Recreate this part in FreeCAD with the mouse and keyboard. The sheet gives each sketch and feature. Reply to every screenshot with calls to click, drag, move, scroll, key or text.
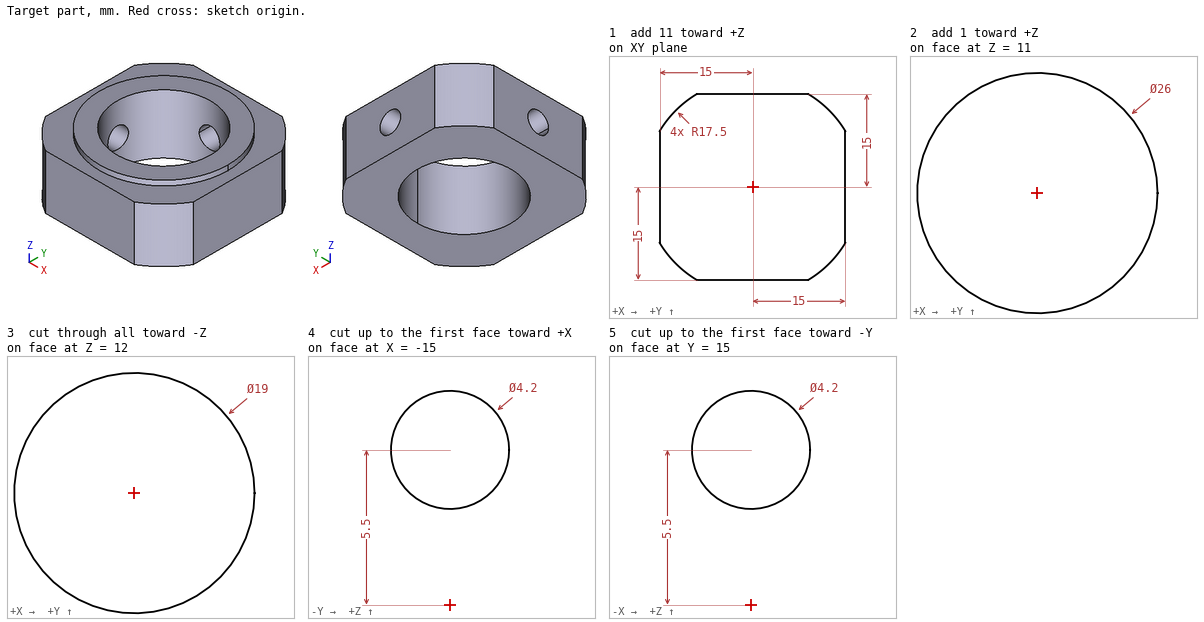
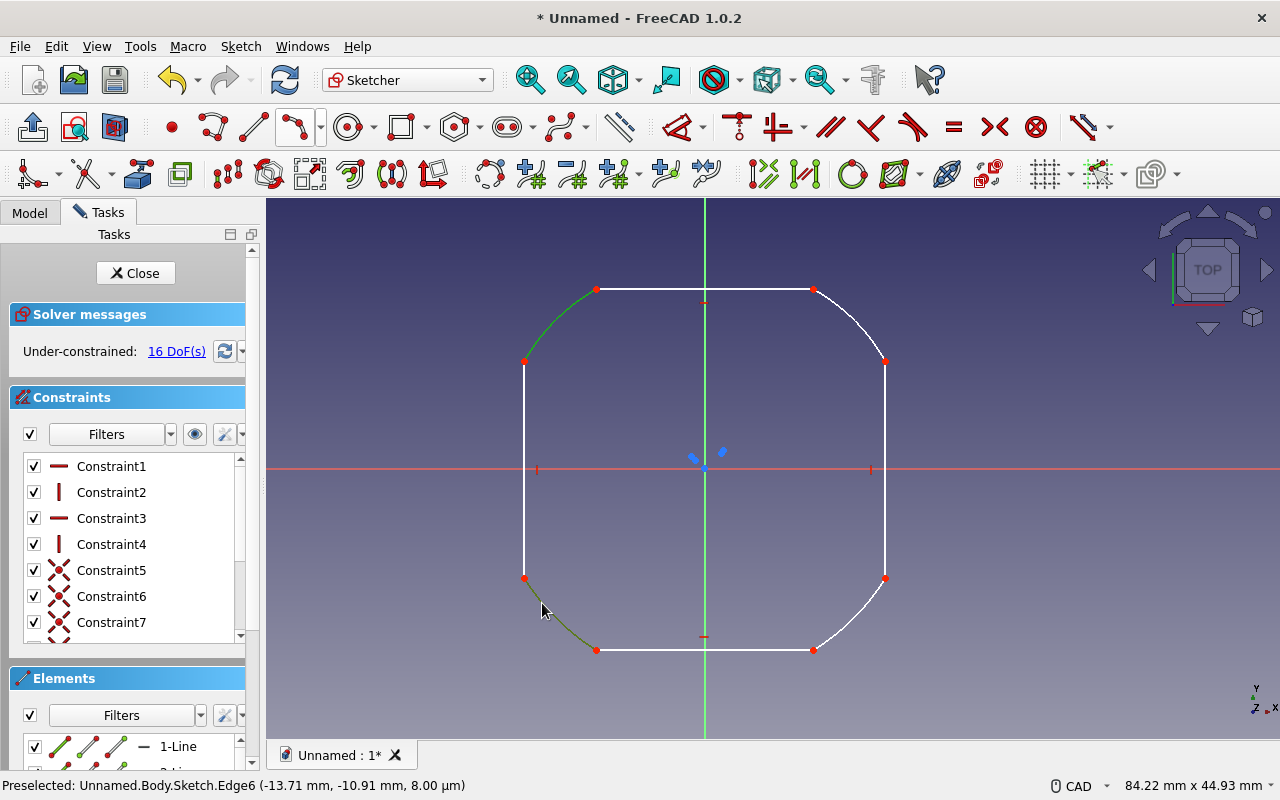
click(737, 128)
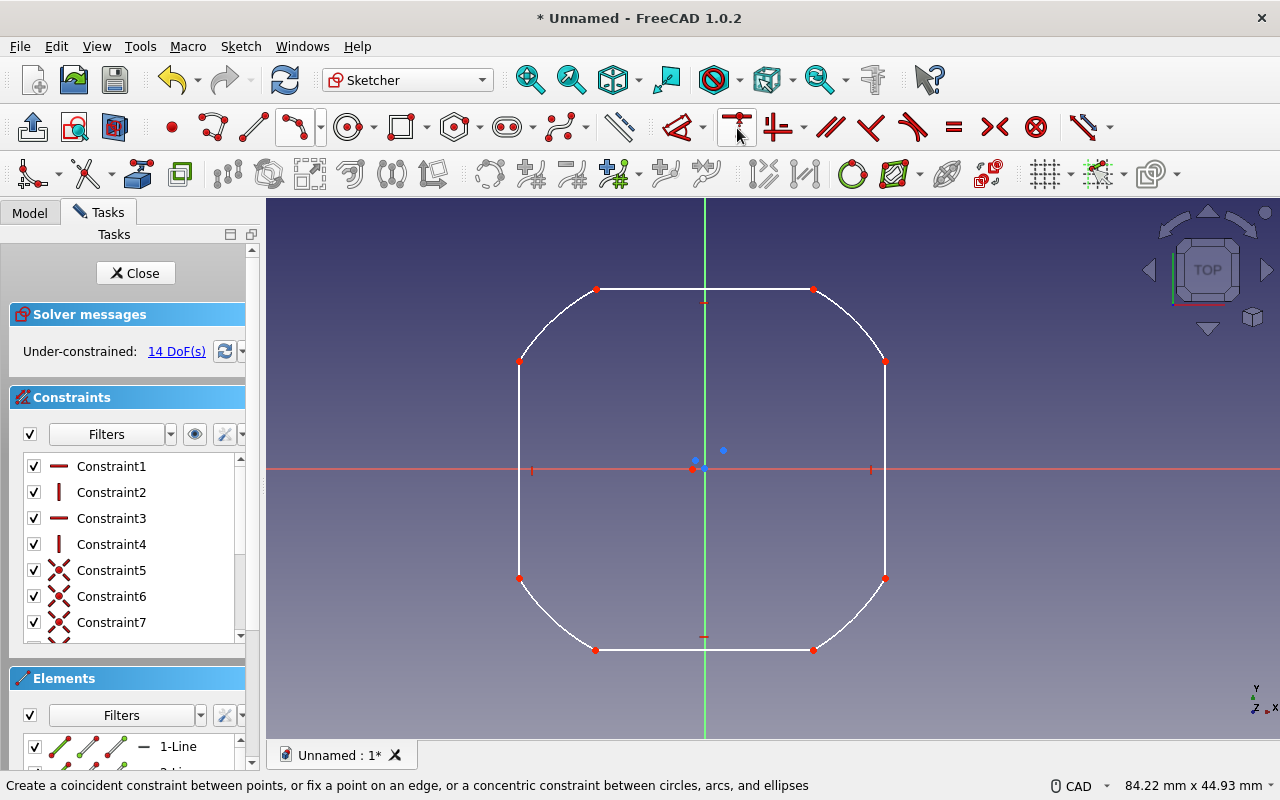
click(569, 306)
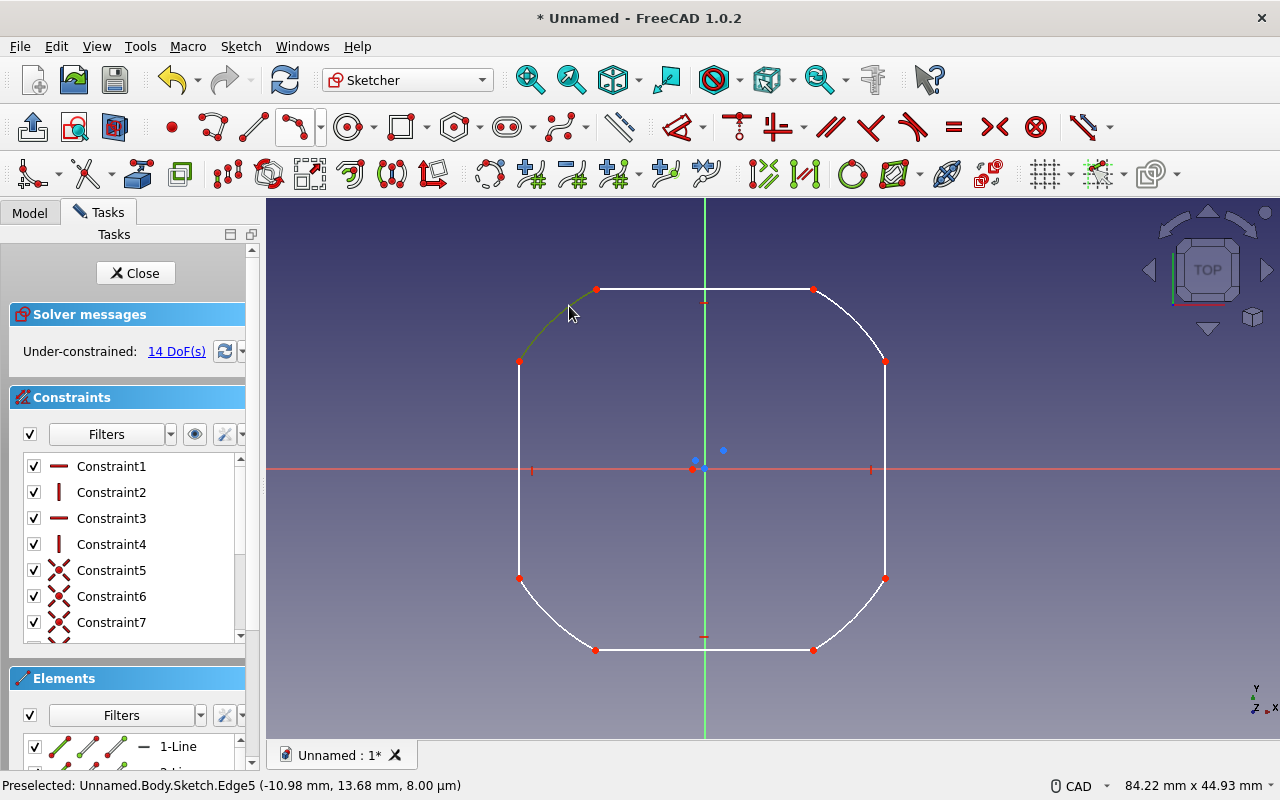
click(838, 632)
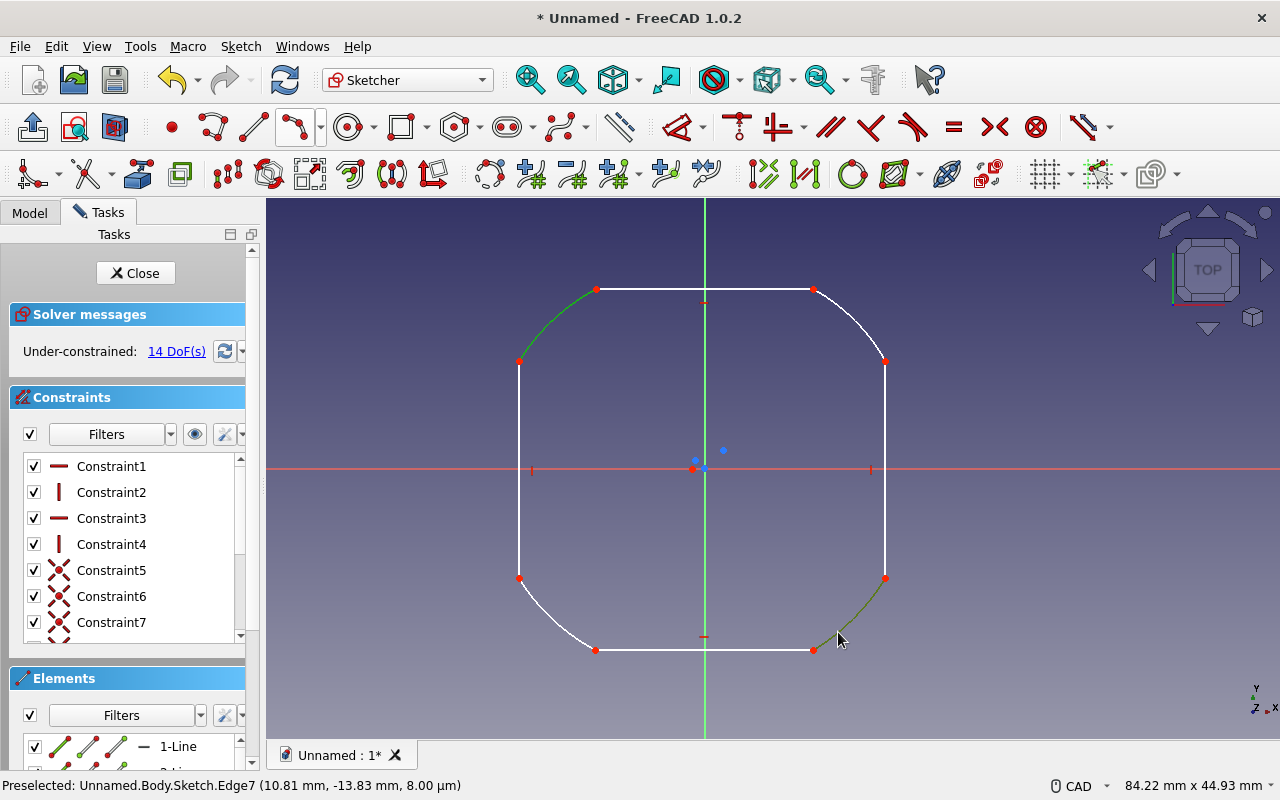
click(737, 128)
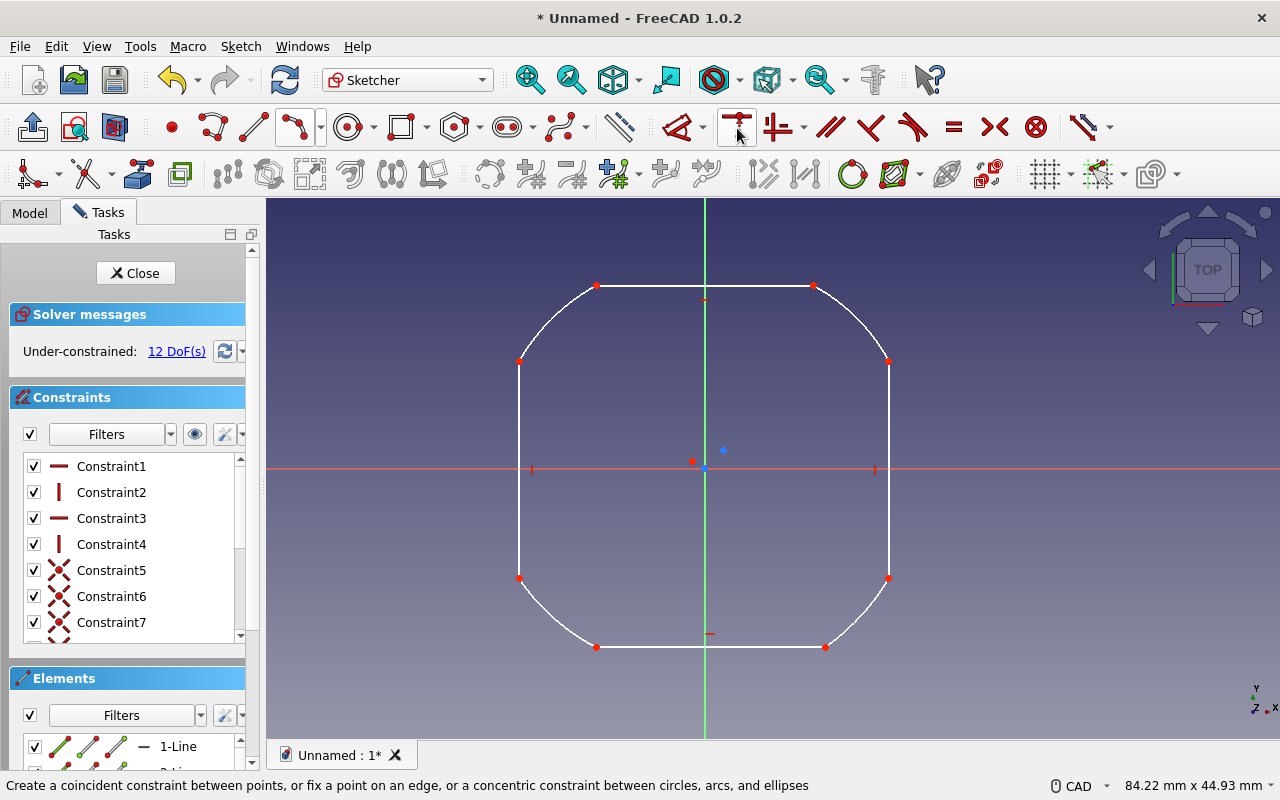
click(569, 304)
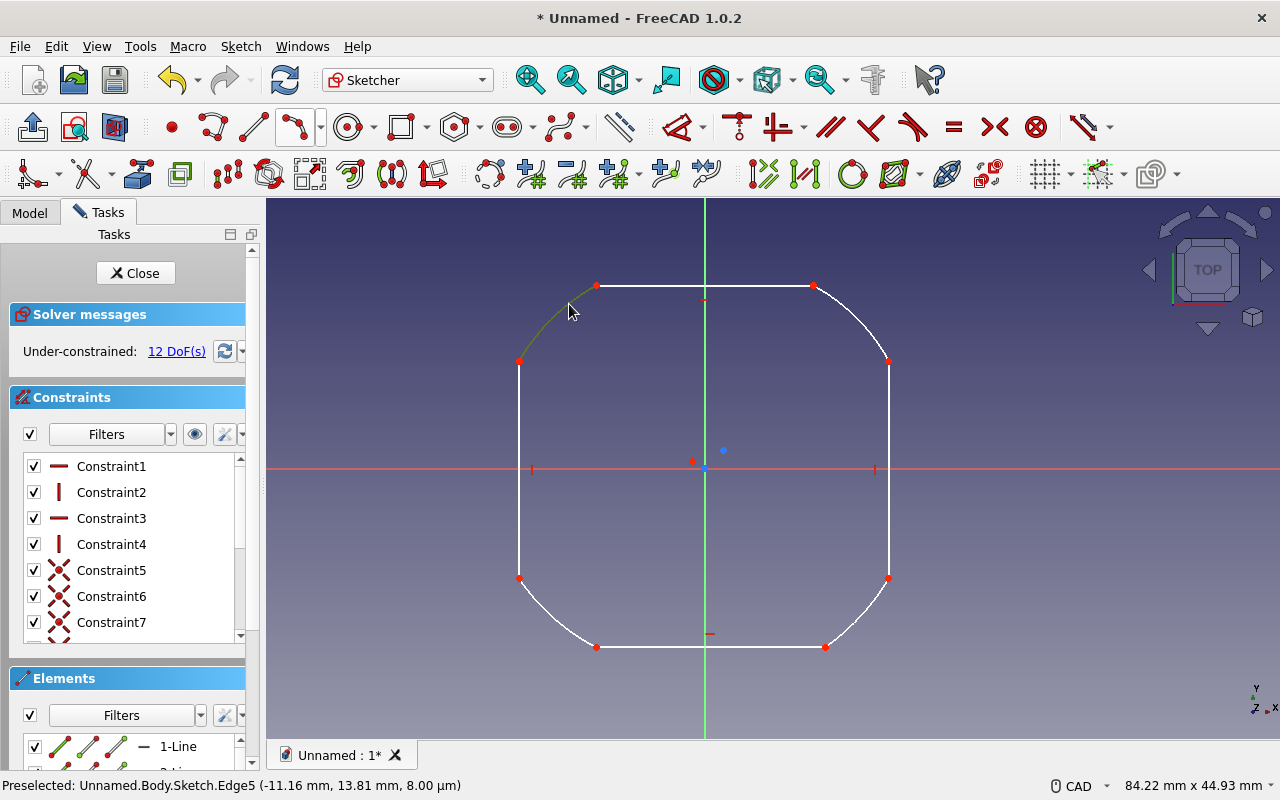
click(871, 334)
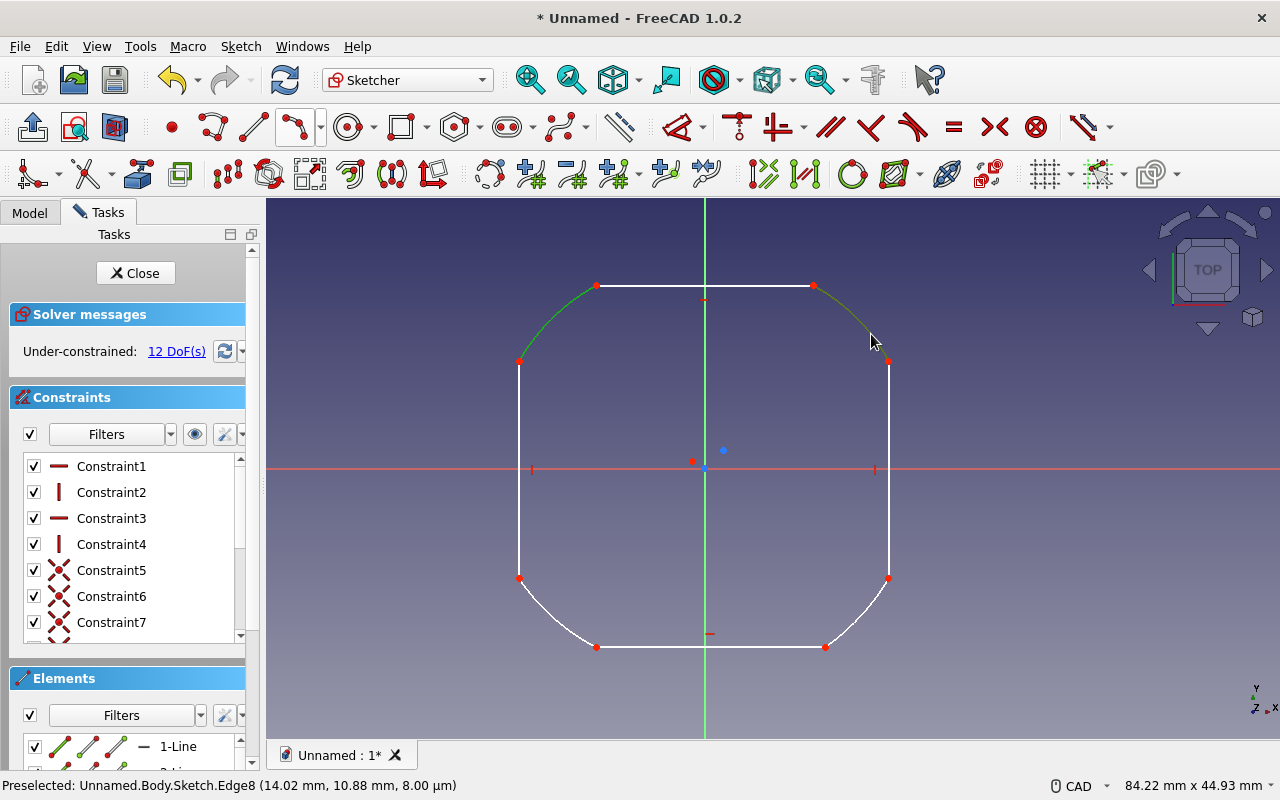
key(c)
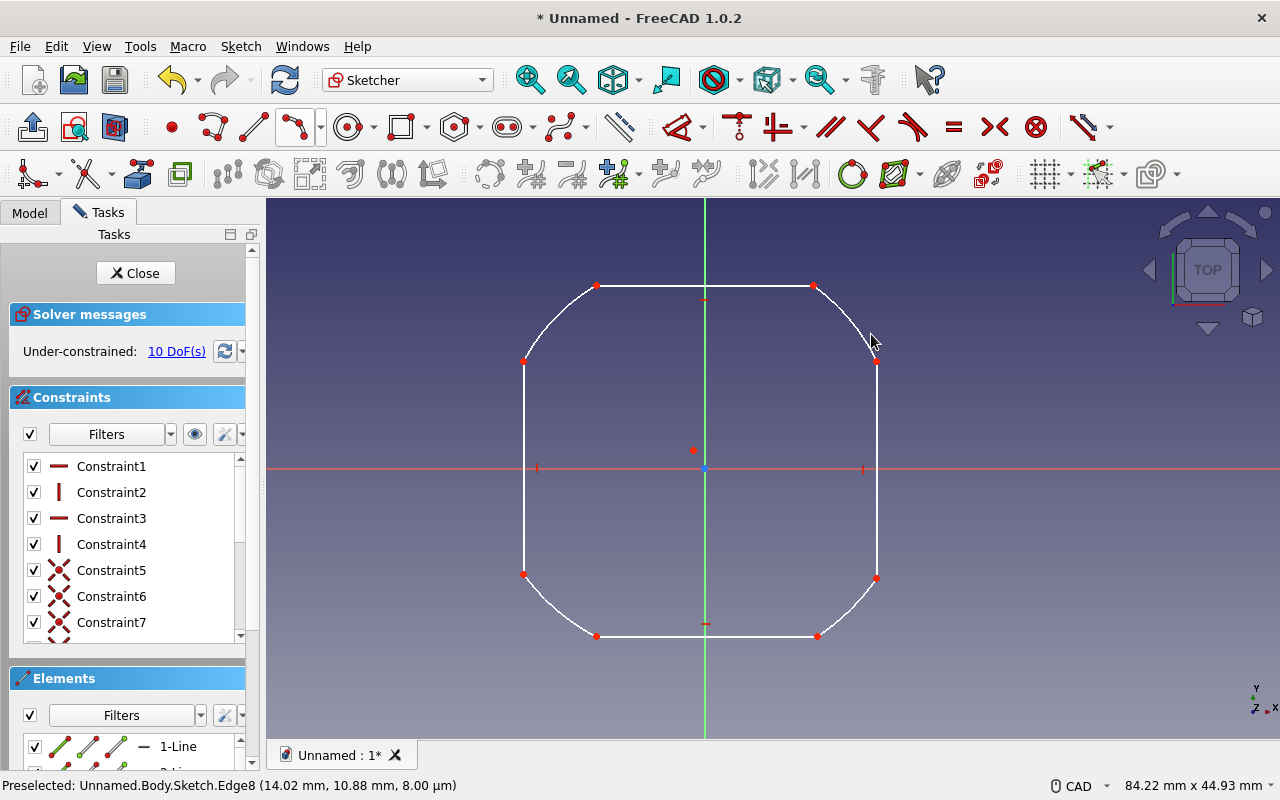
drag(683, 441, 715, 479)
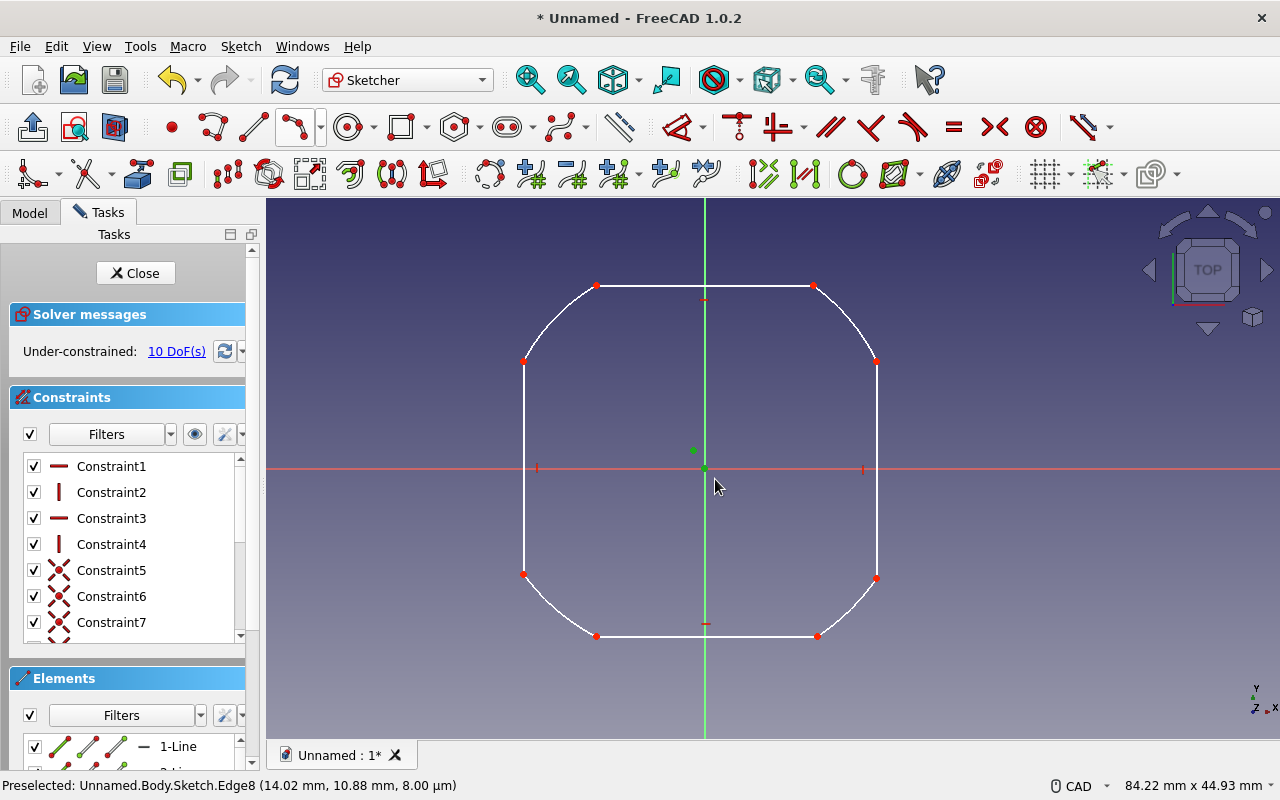
click(737, 128)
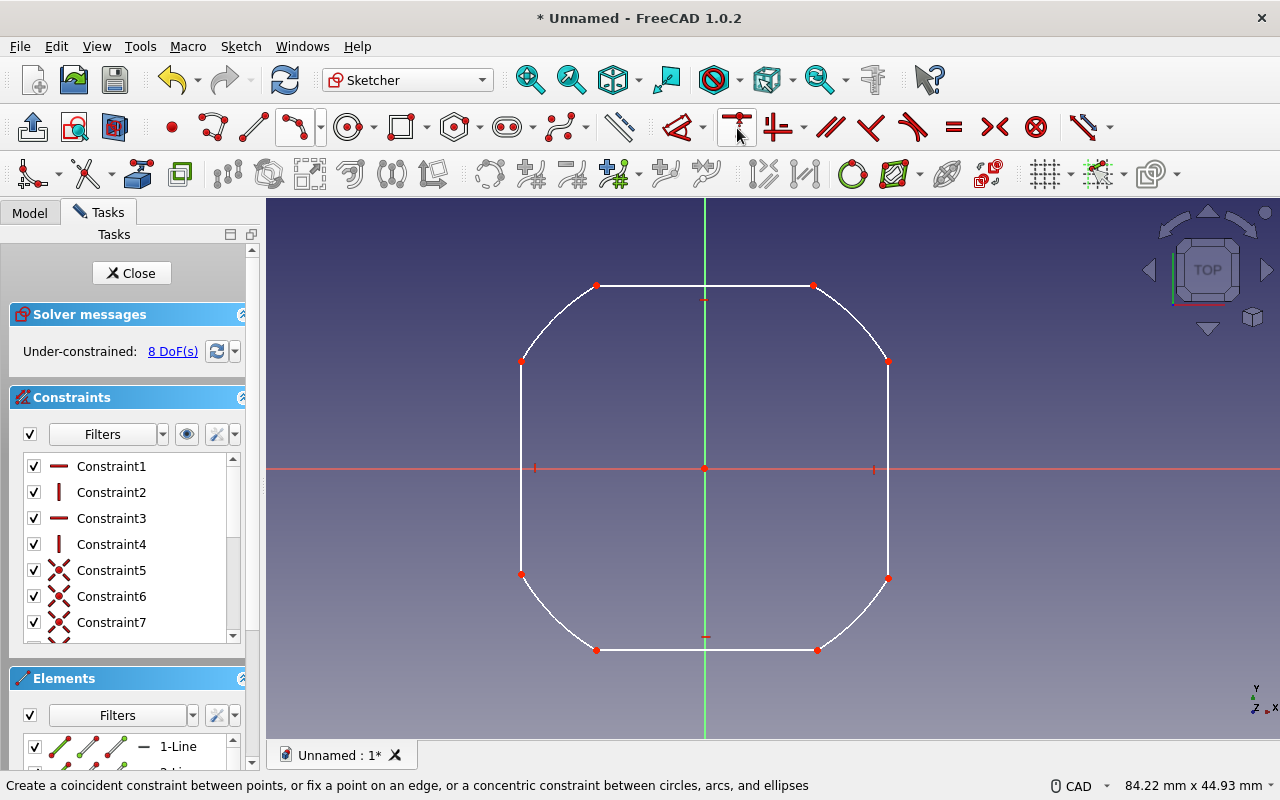
click(570, 304)